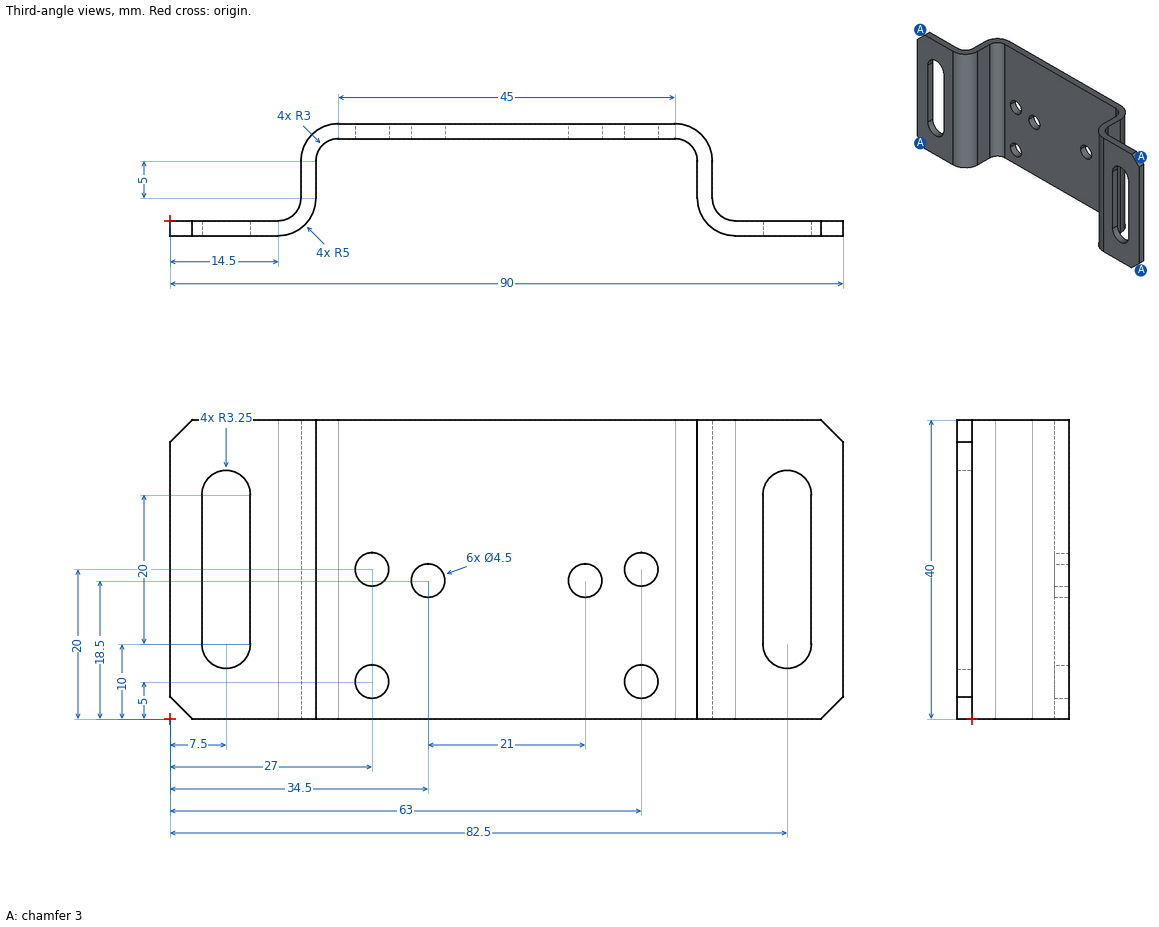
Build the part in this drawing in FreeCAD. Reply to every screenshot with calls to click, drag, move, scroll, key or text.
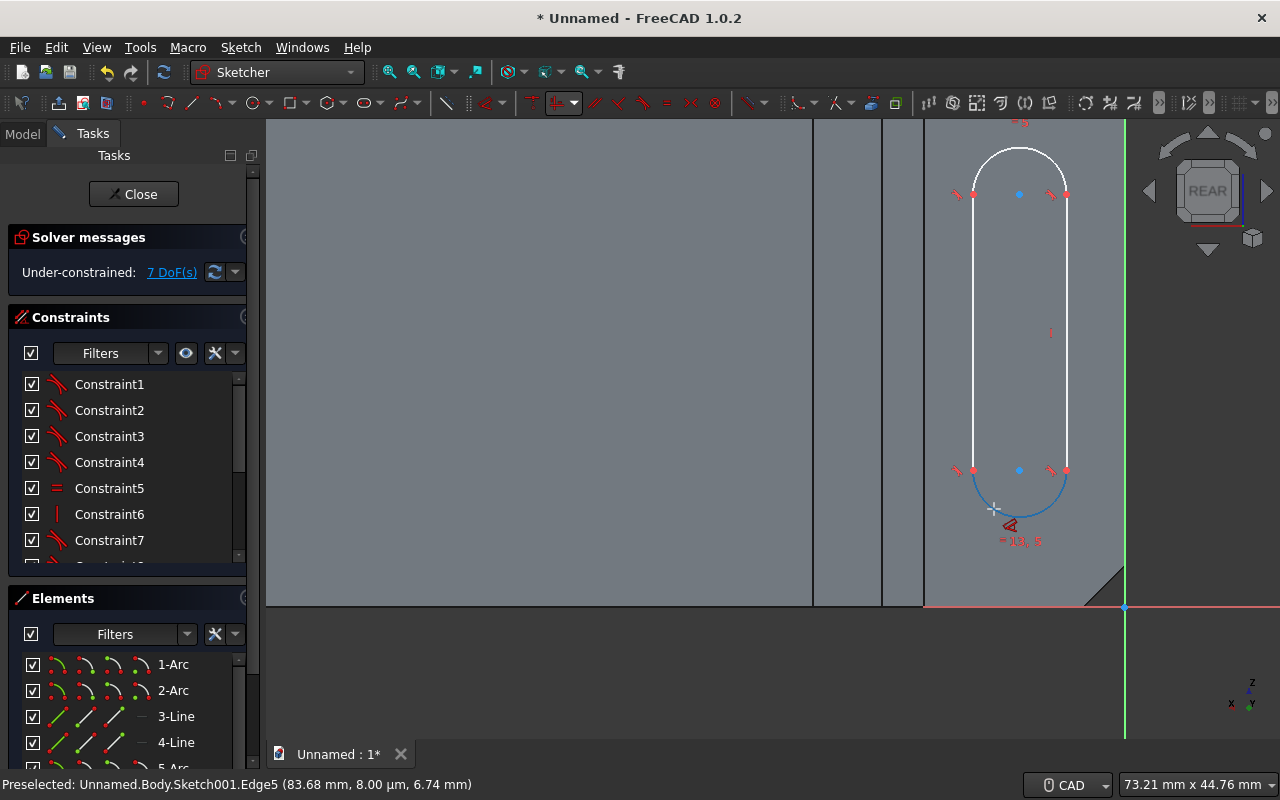
click(992, 508)
click(973, 534)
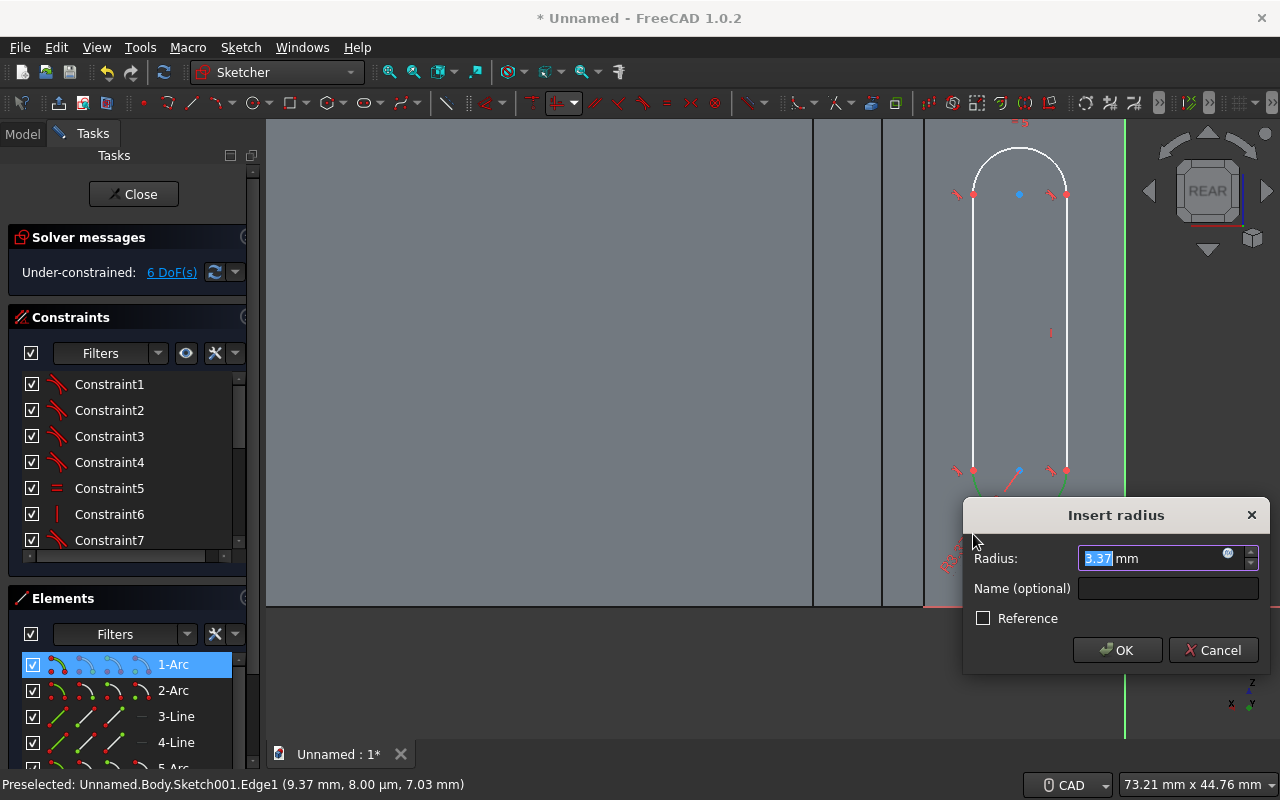
text(3.25)
key(Return)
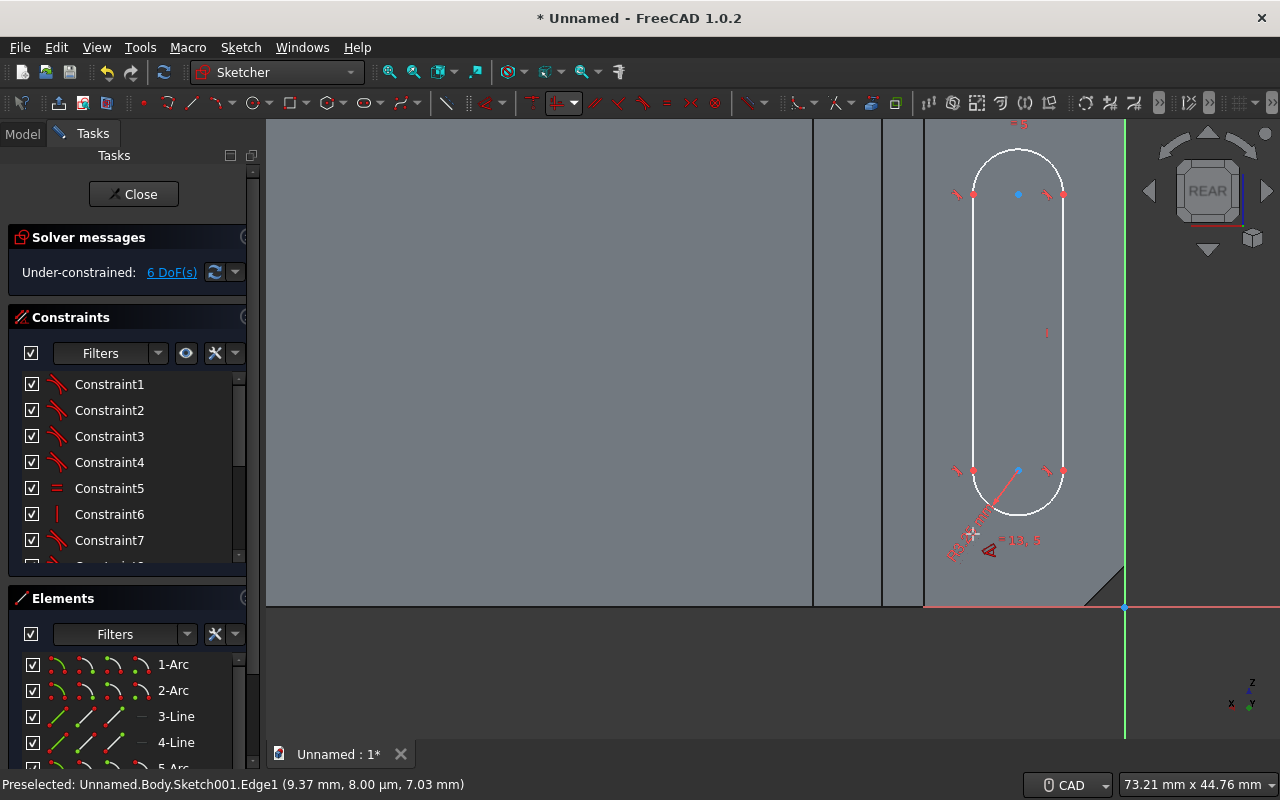
click(973, 388)
click(1007, 332)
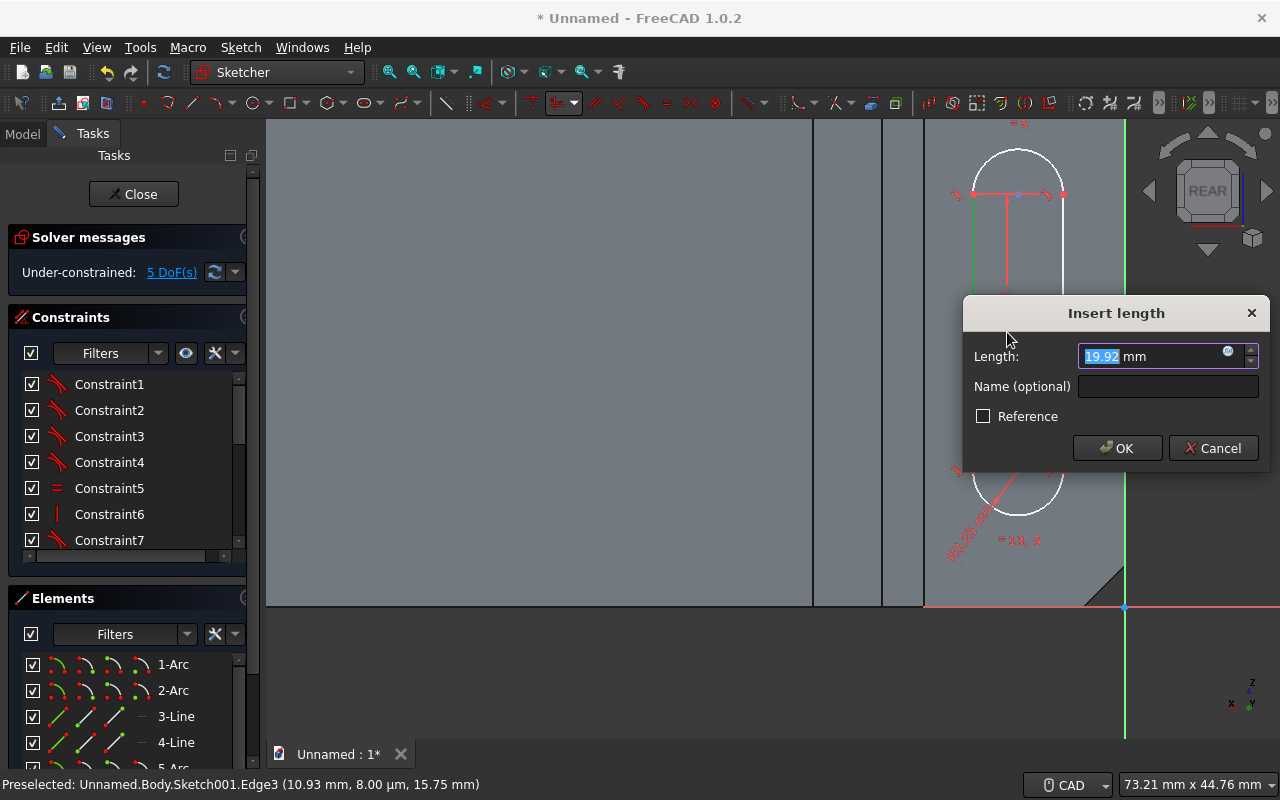
text(20)
key(Return)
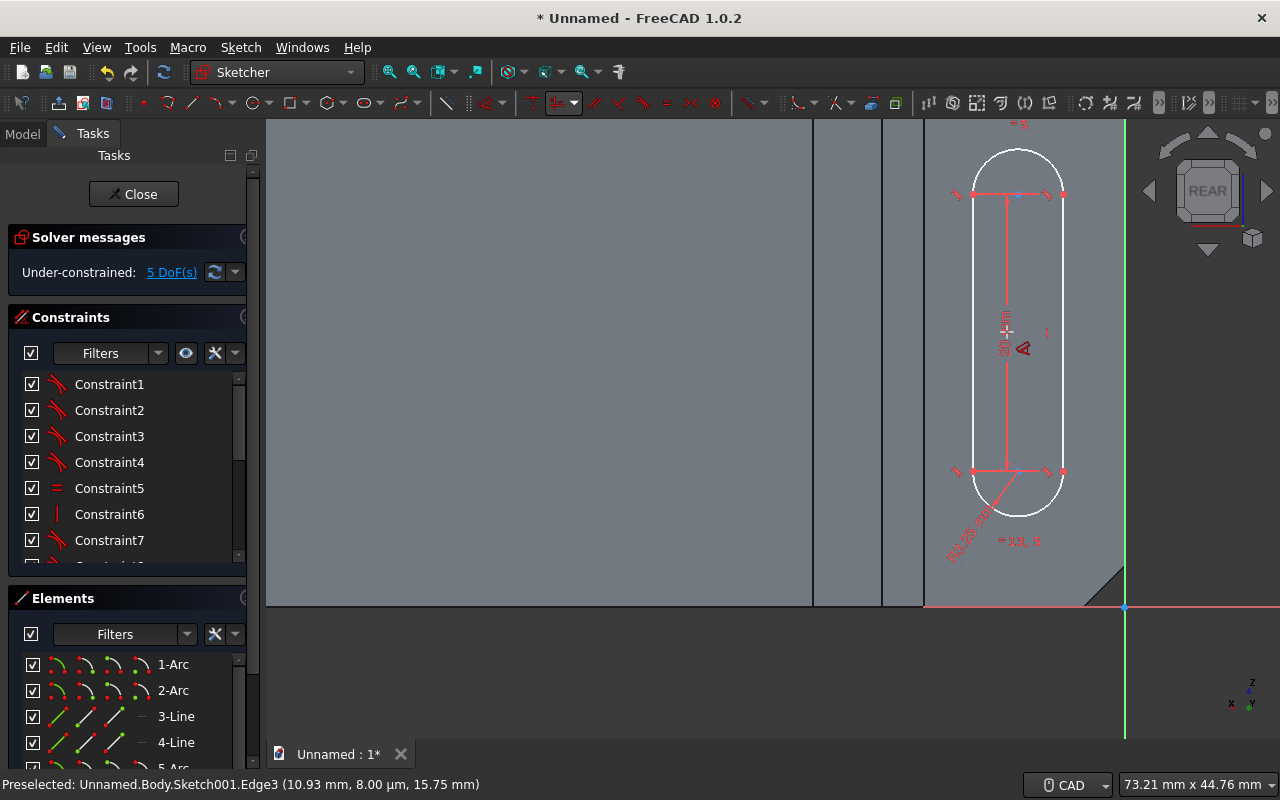
scroll(846, 471, down, 4)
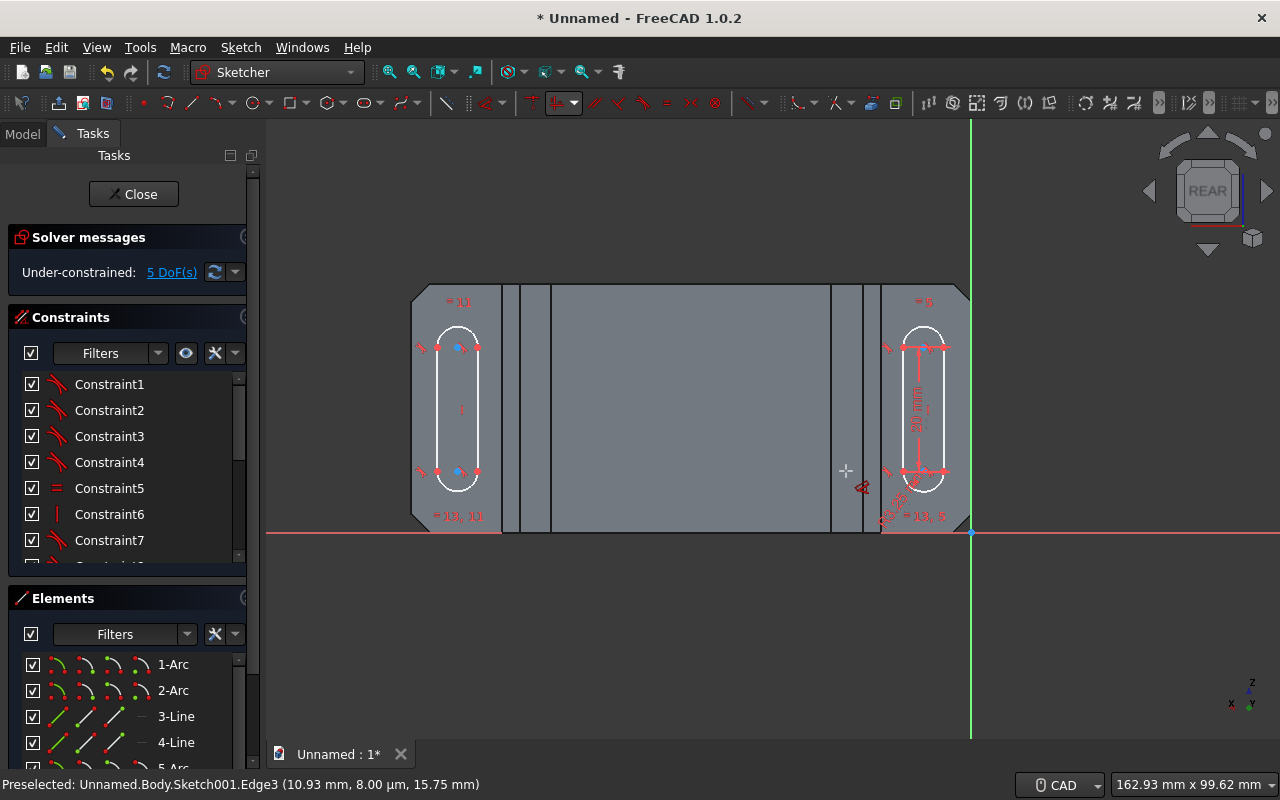
click(437, 434)
click(403, 409)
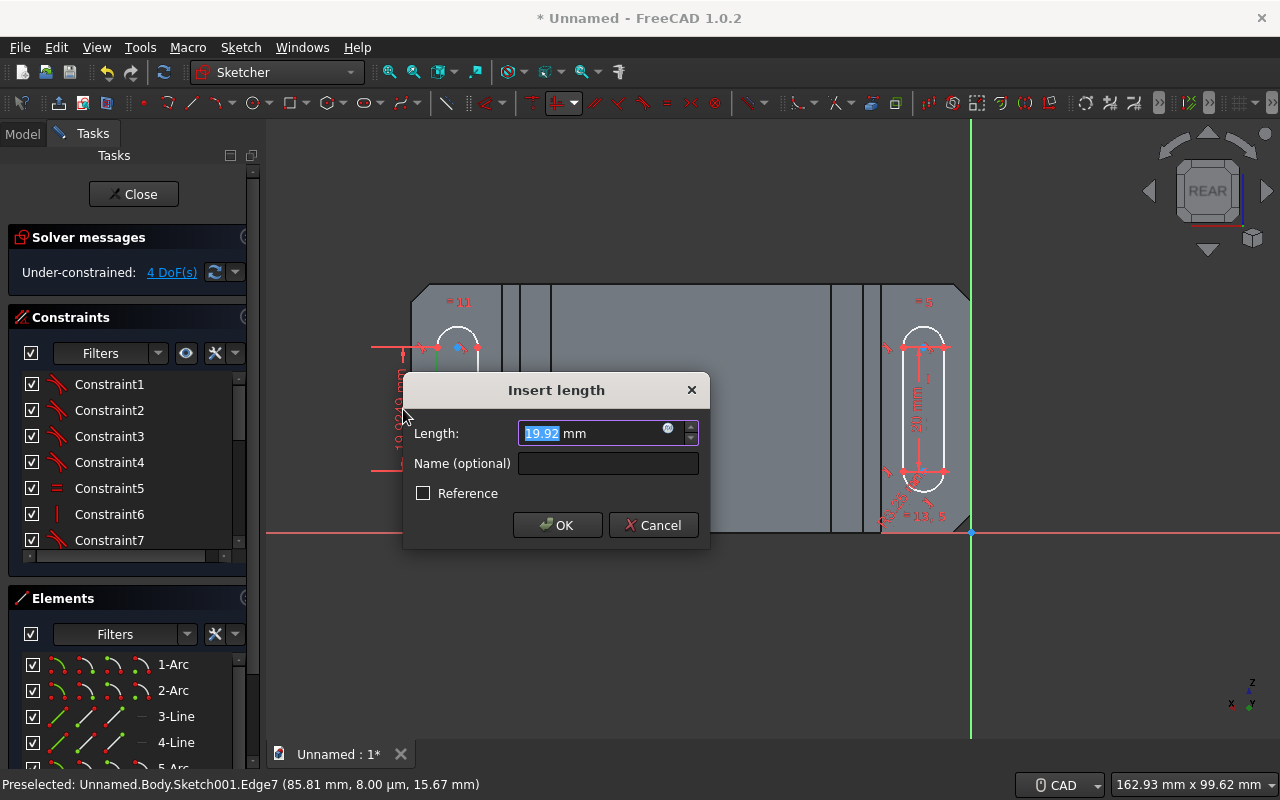
text(20)
key(Return)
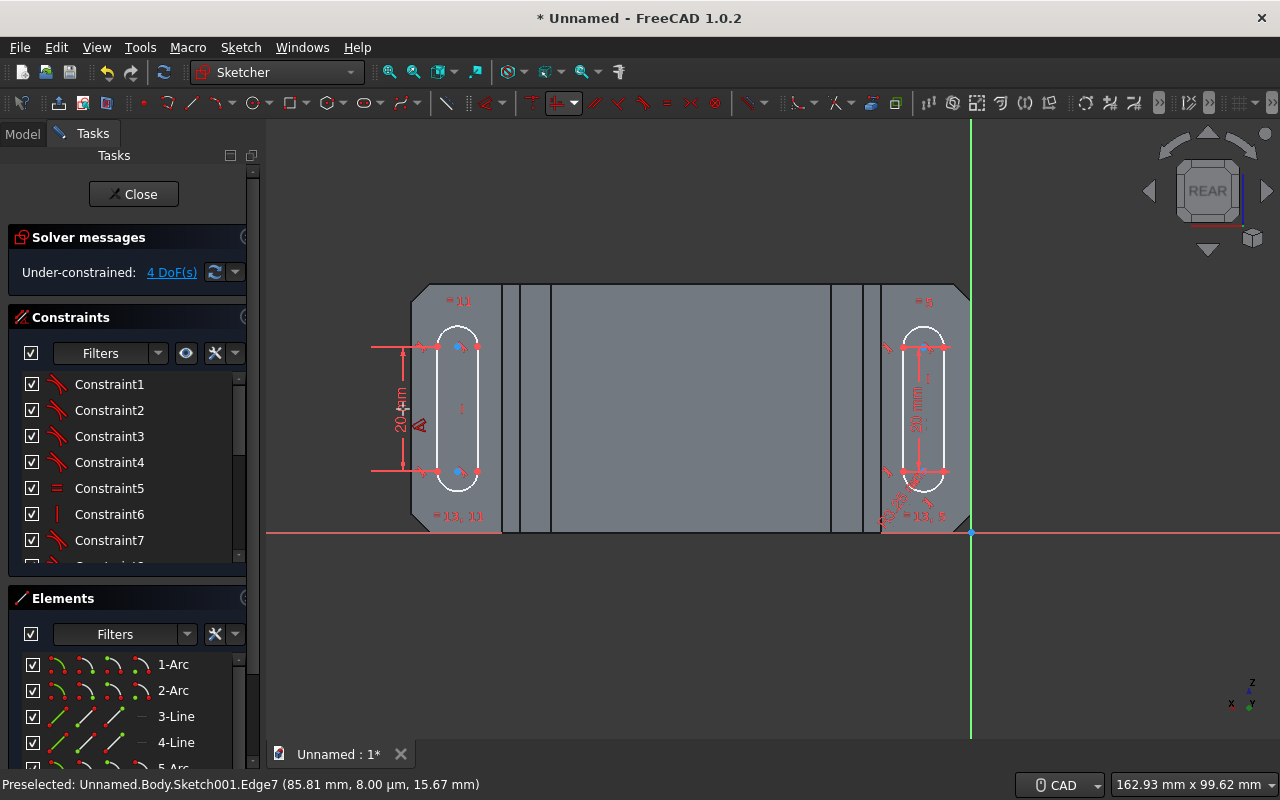
click(903, 472)
click(1005, 502)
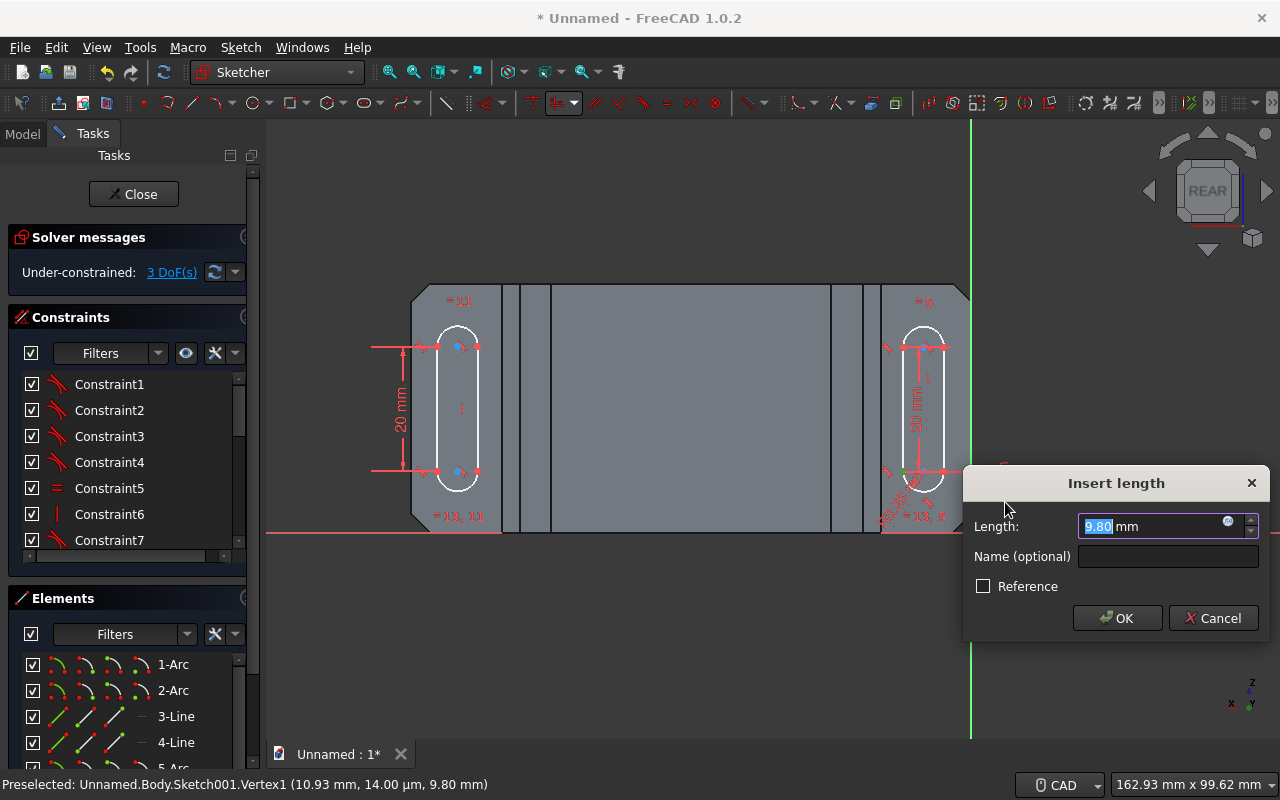
text(10)
key(Return)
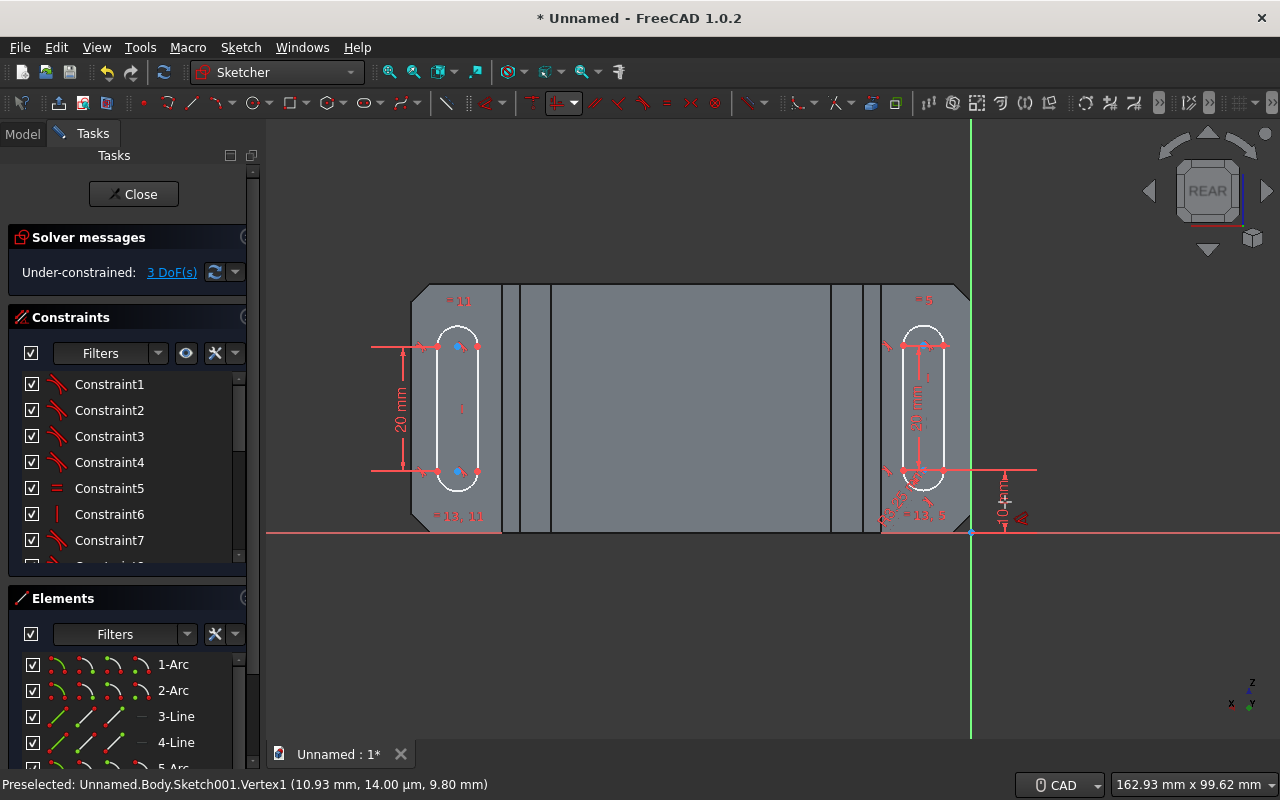
click(437, 471)
click(403, 502)